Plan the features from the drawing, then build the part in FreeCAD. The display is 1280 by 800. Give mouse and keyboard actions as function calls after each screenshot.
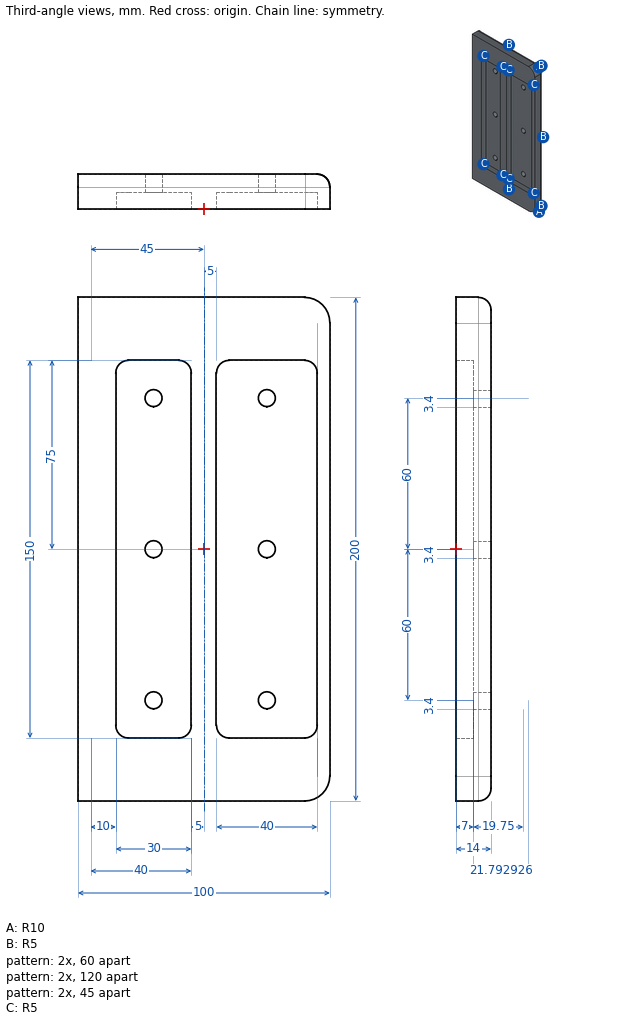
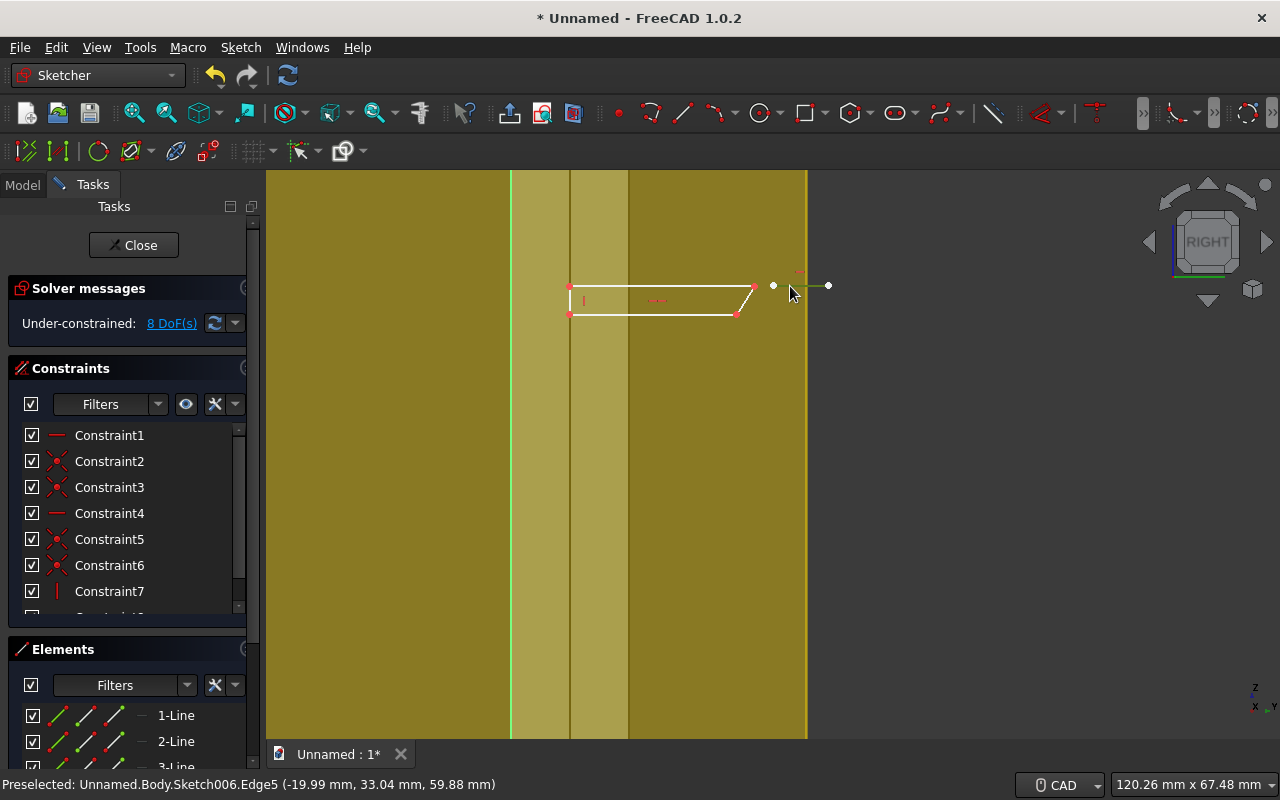
click(994, 114)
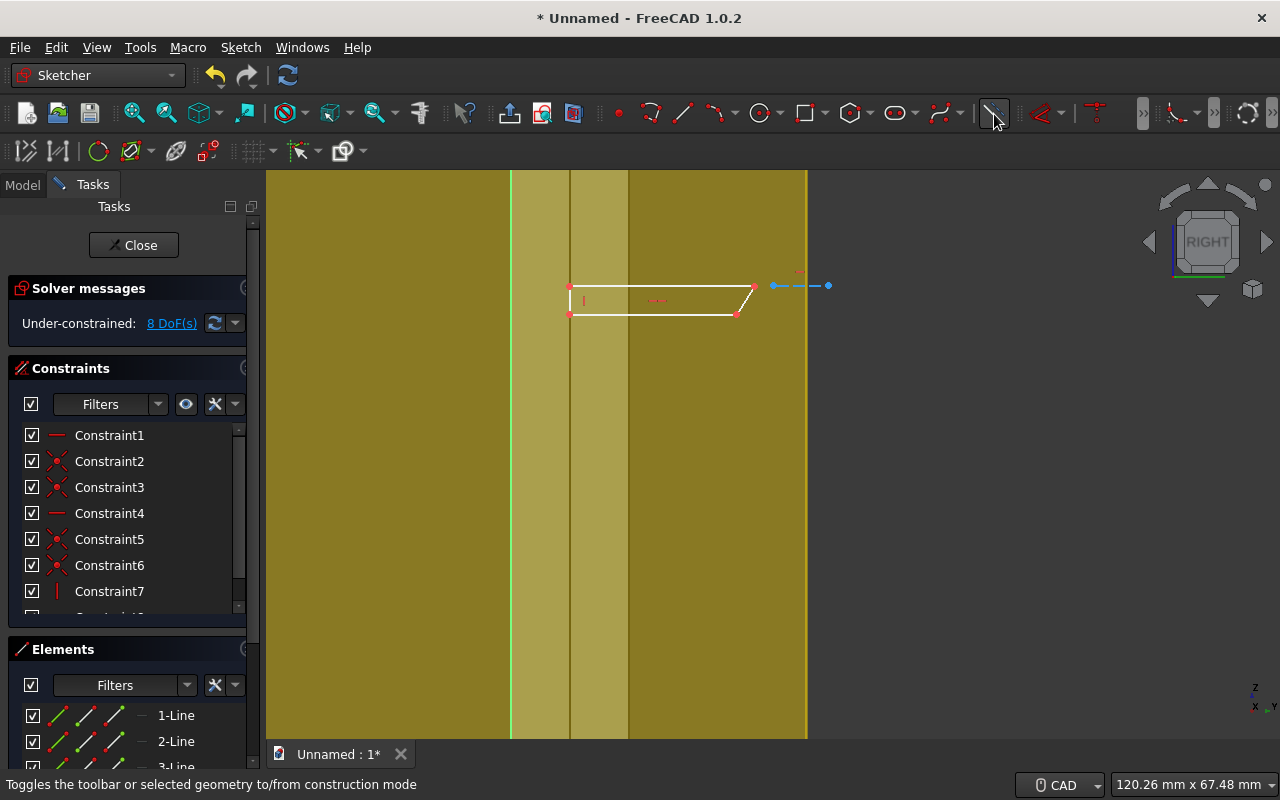
click(1040, 114)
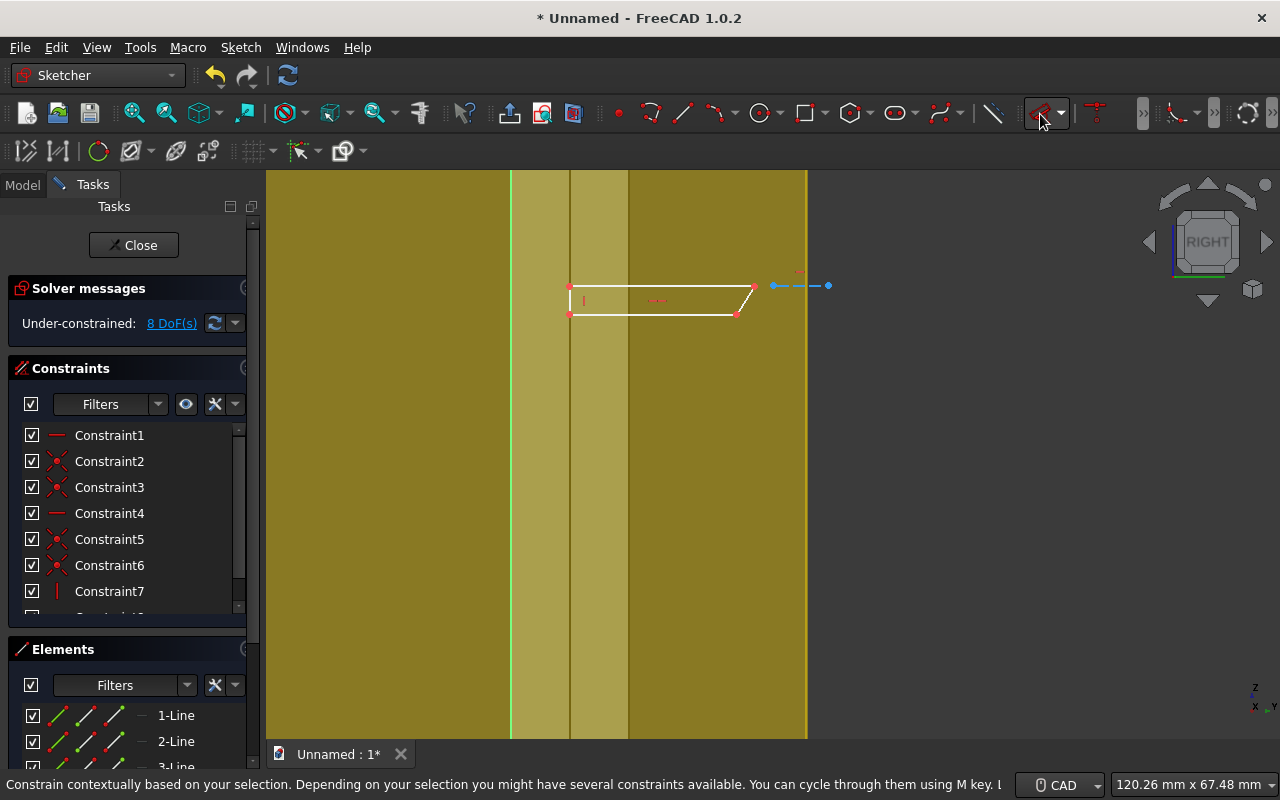
click(570, 315)
click(541, 281)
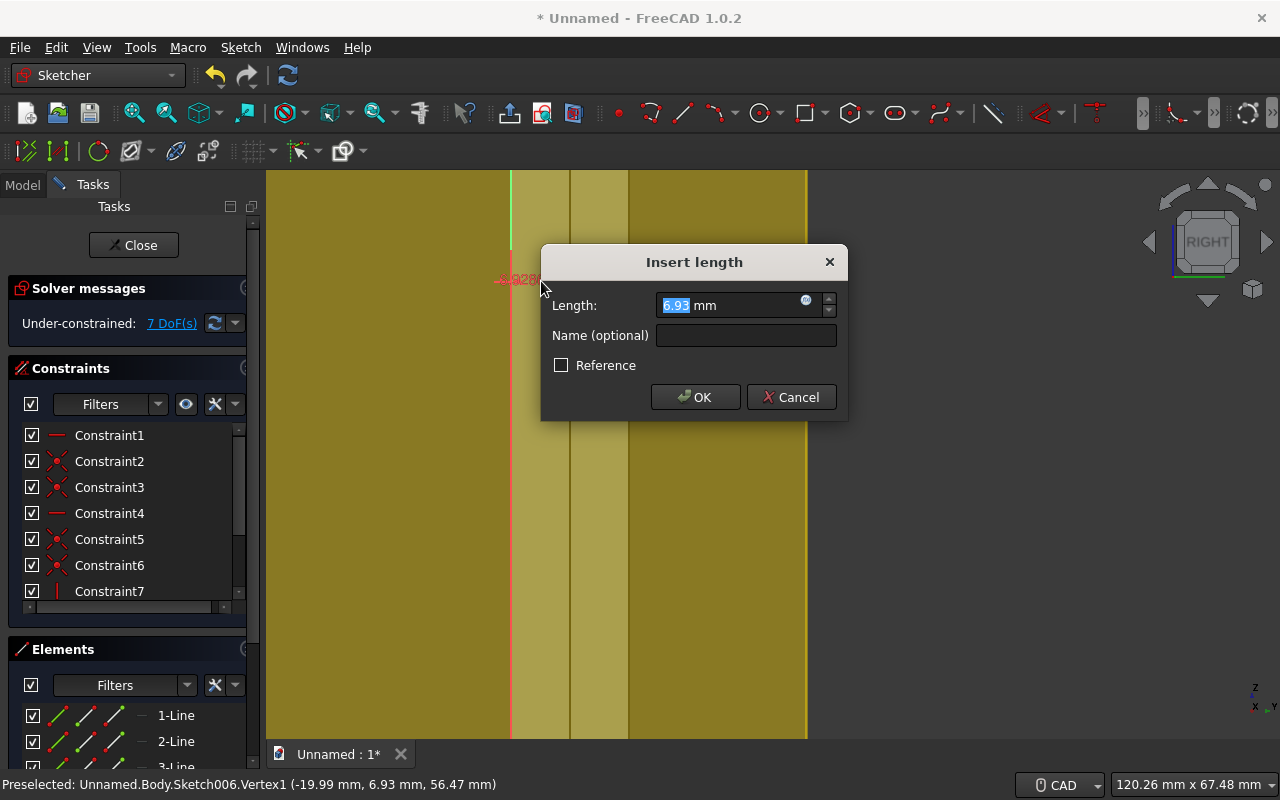
text(7)
key(Return)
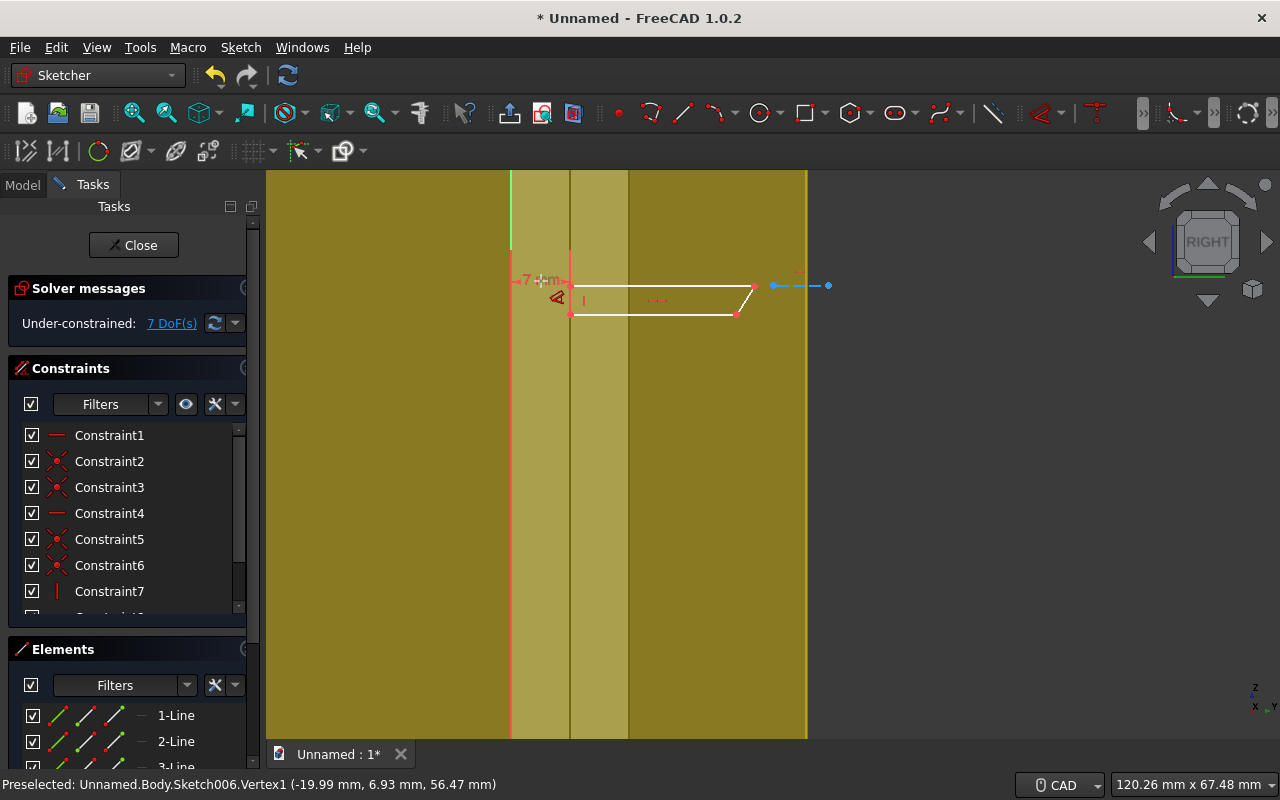
scroll(570, 298, up, 2)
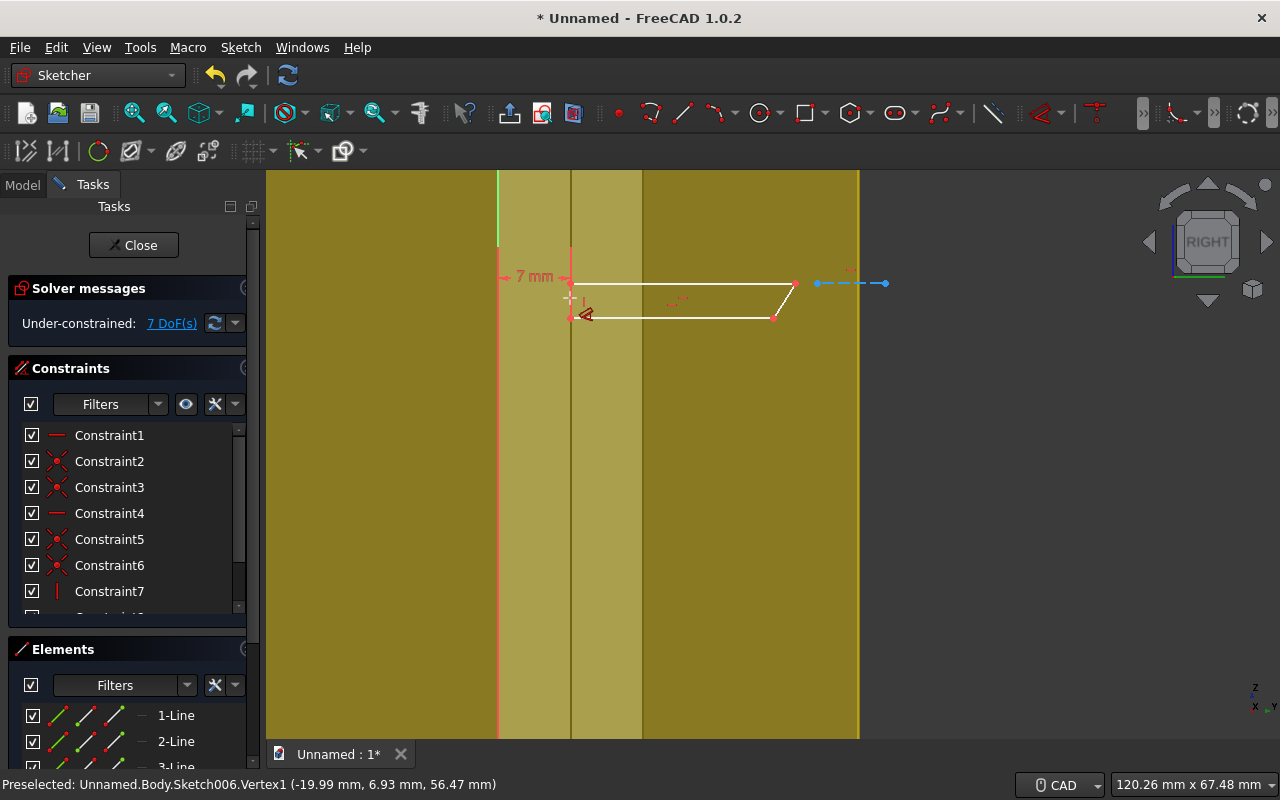
click(571, 297)
click(537, 302)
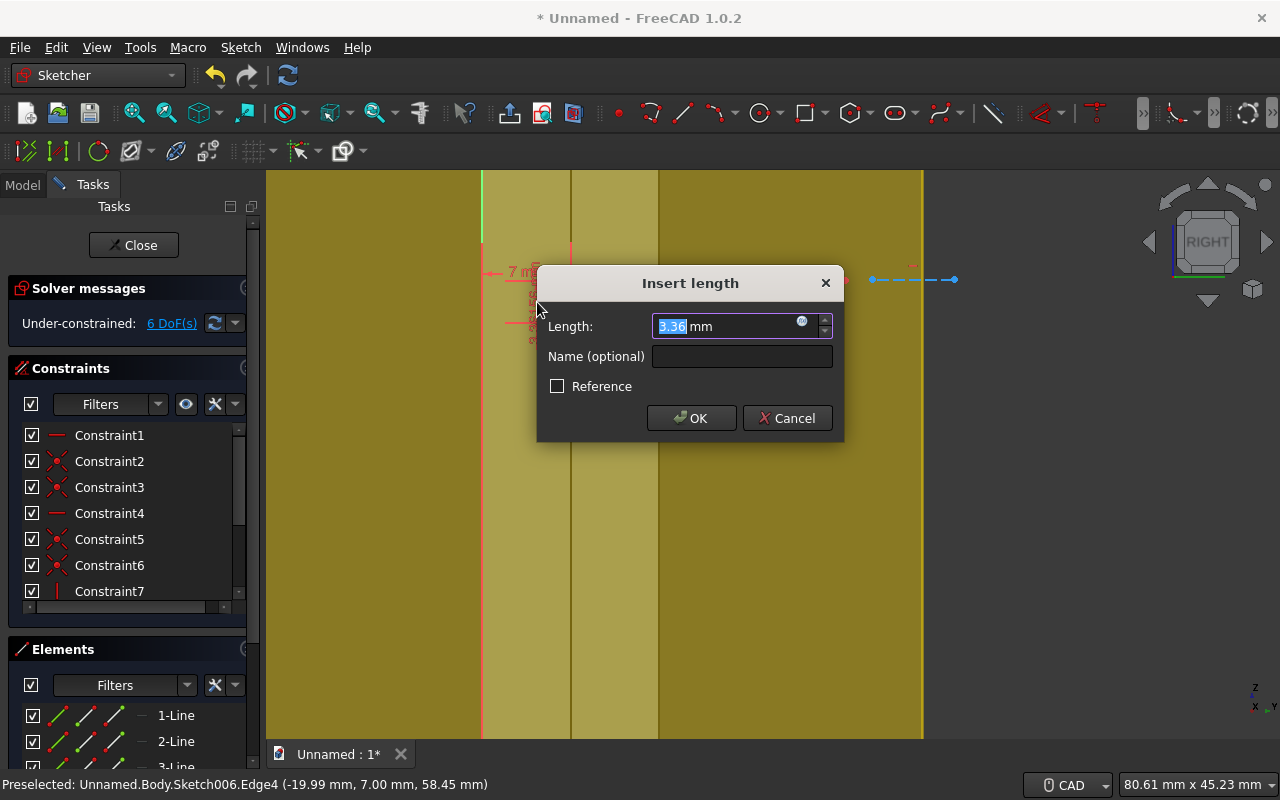
text(3.4)
key(Return)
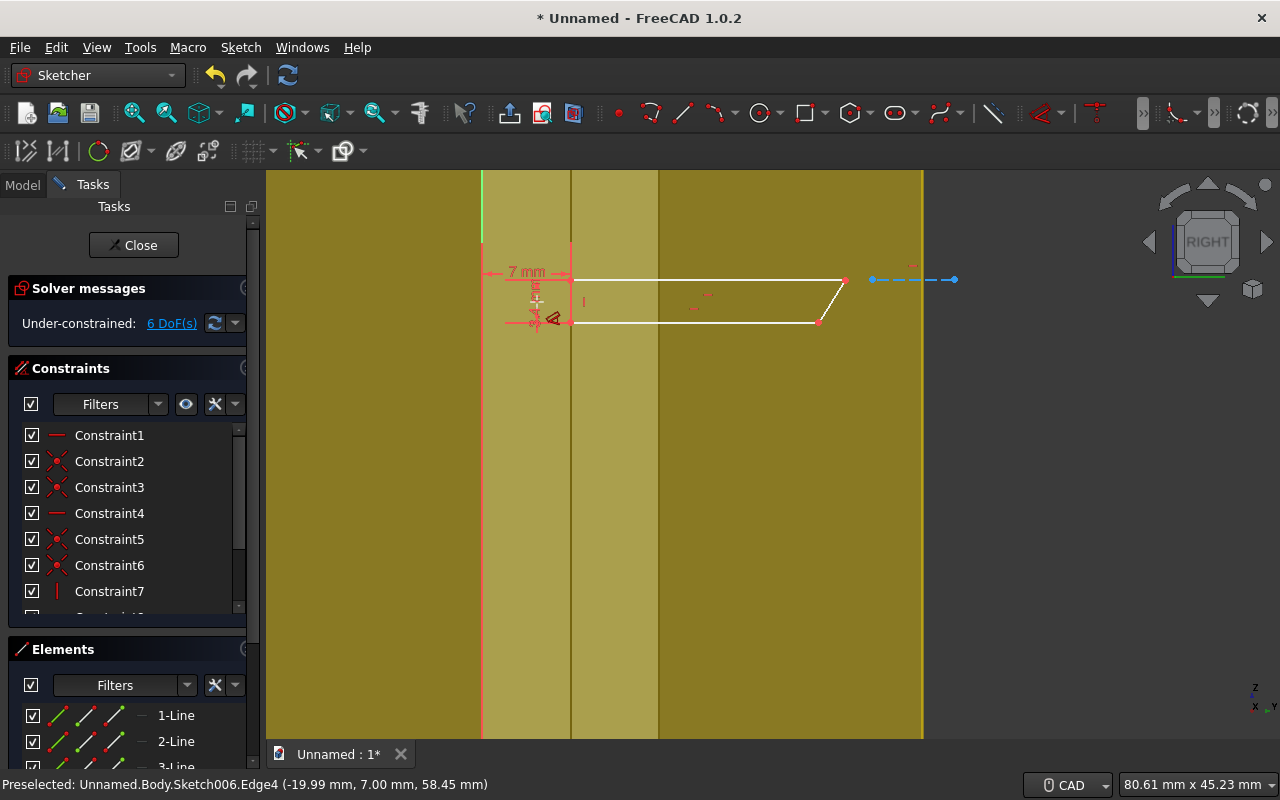
click(846, 280)
click(448, 496)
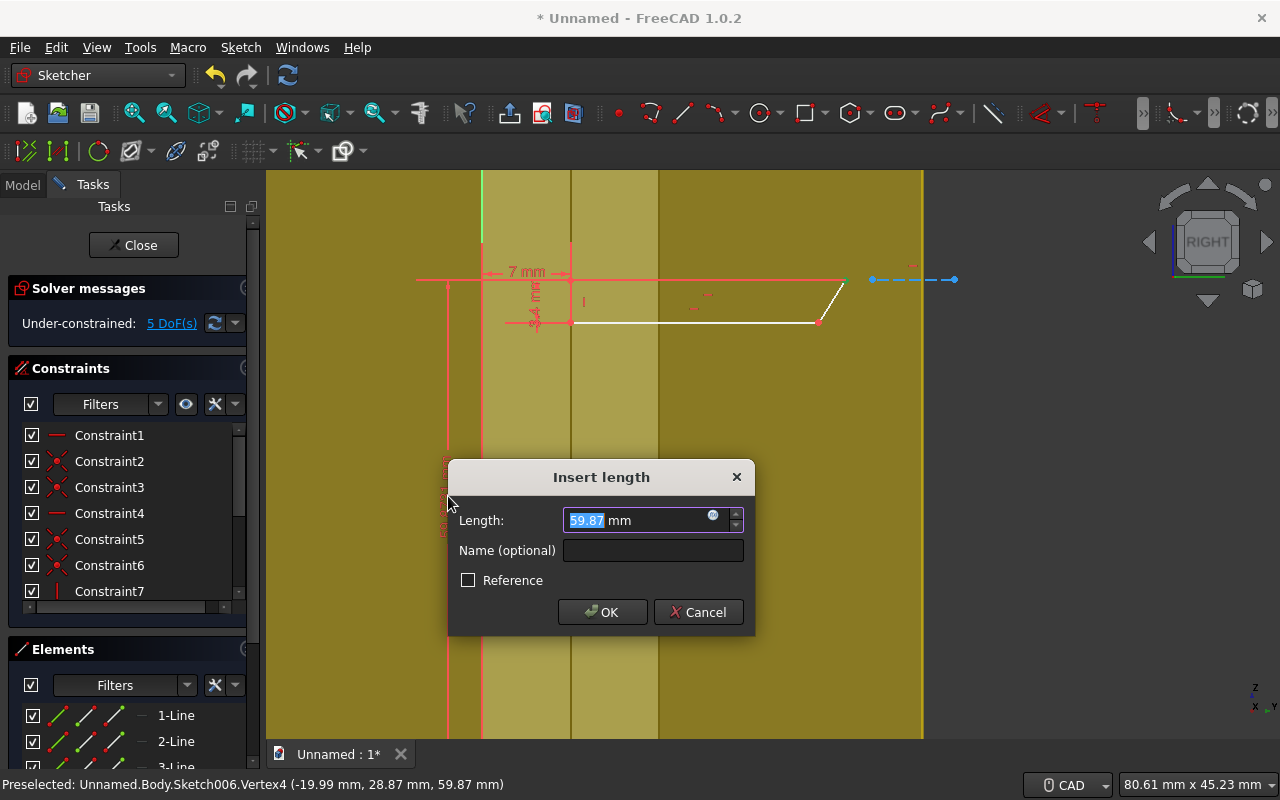
text(60)
key(Return)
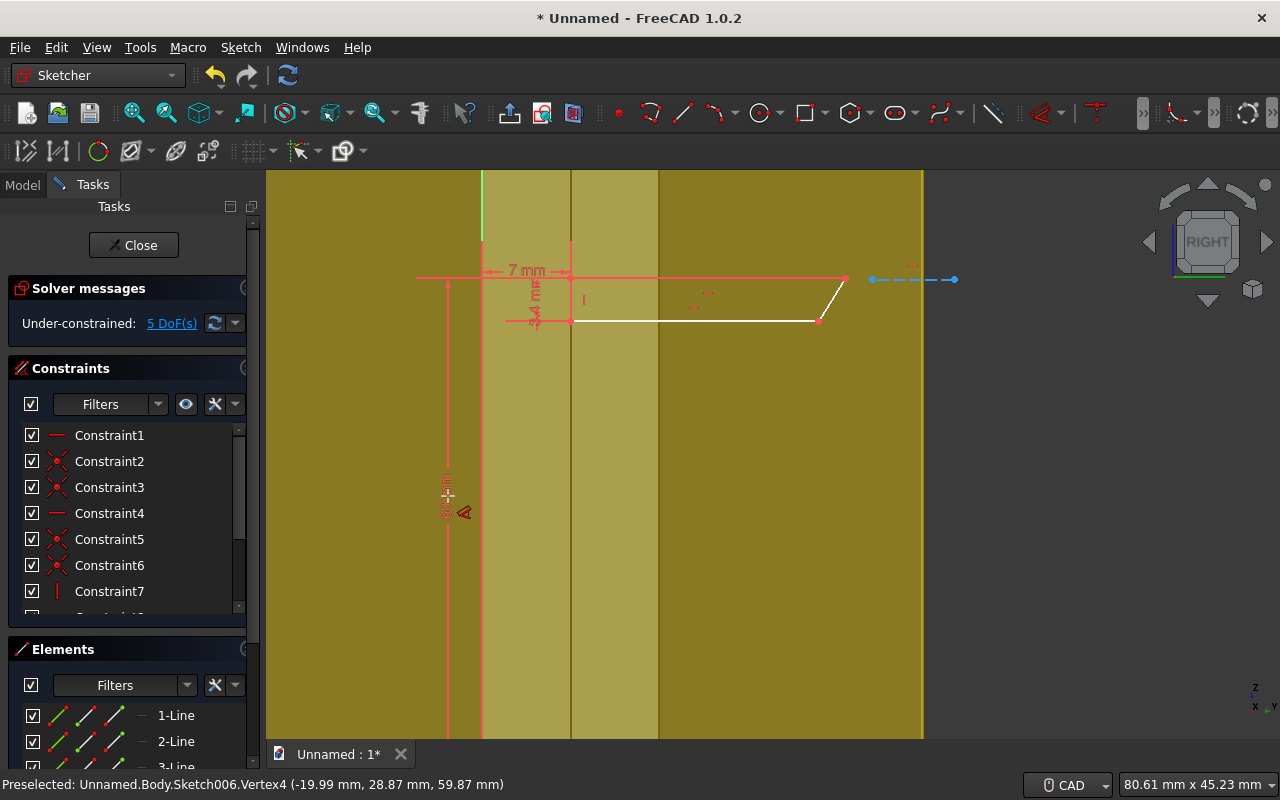
click(873, 280)
click(448, 396)